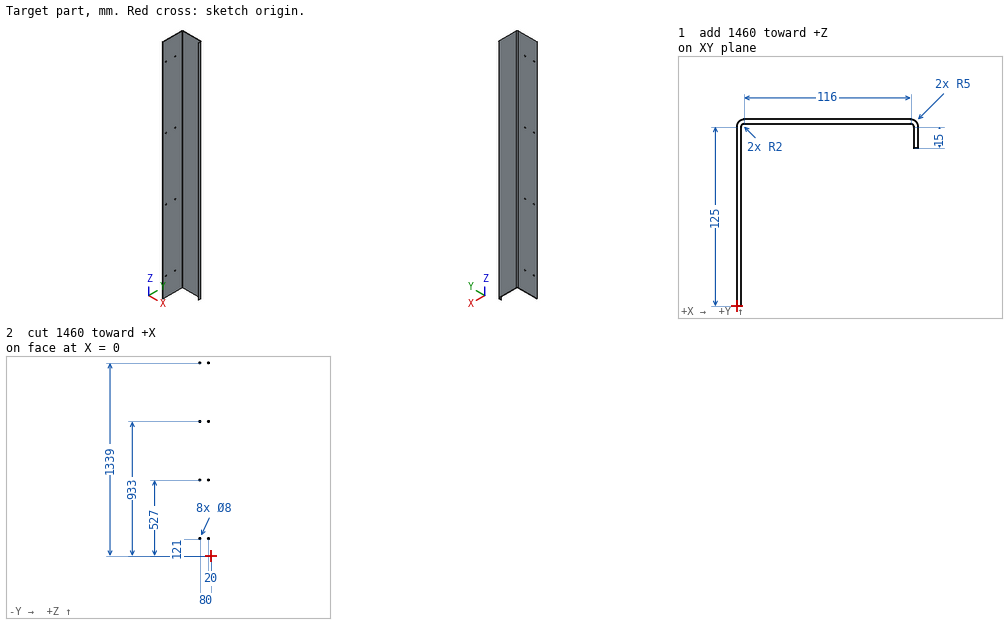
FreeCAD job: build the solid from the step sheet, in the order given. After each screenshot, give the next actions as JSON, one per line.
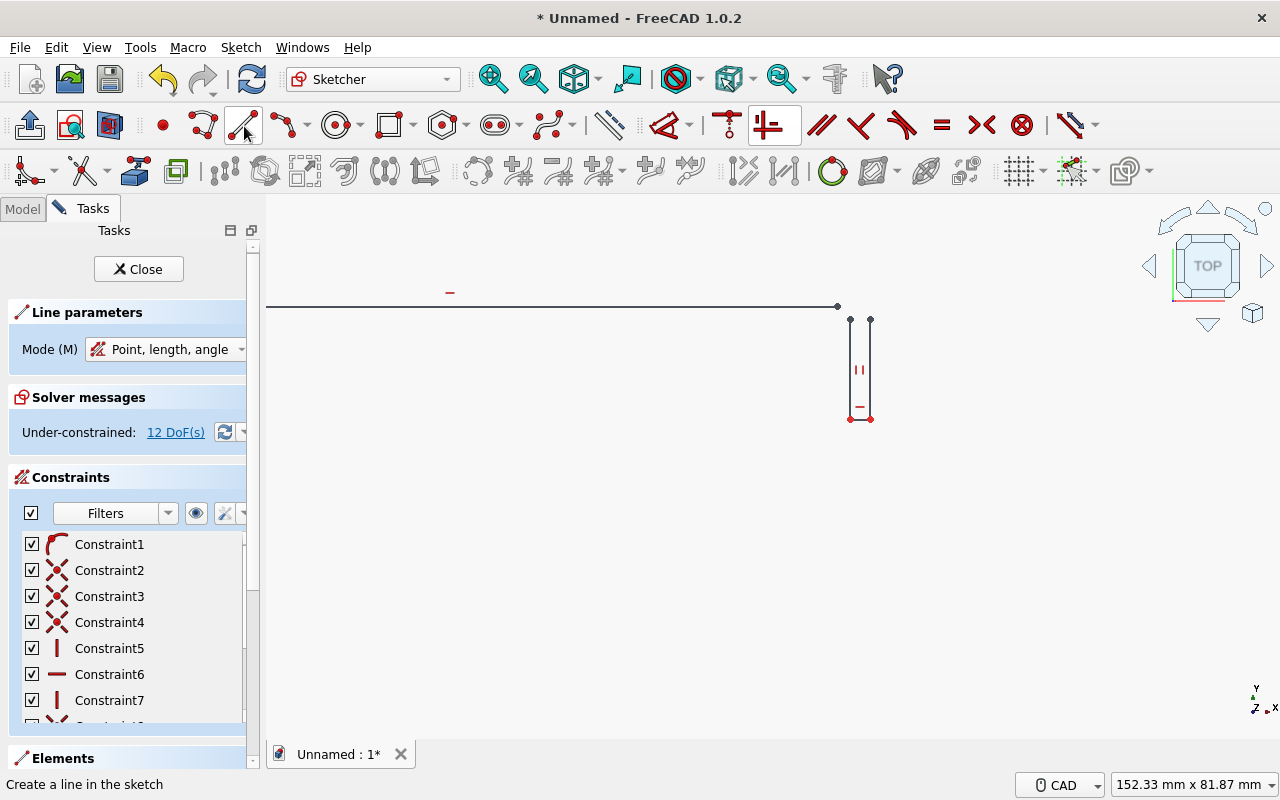
{"action": "left_click", "coordinate": [837, 286]}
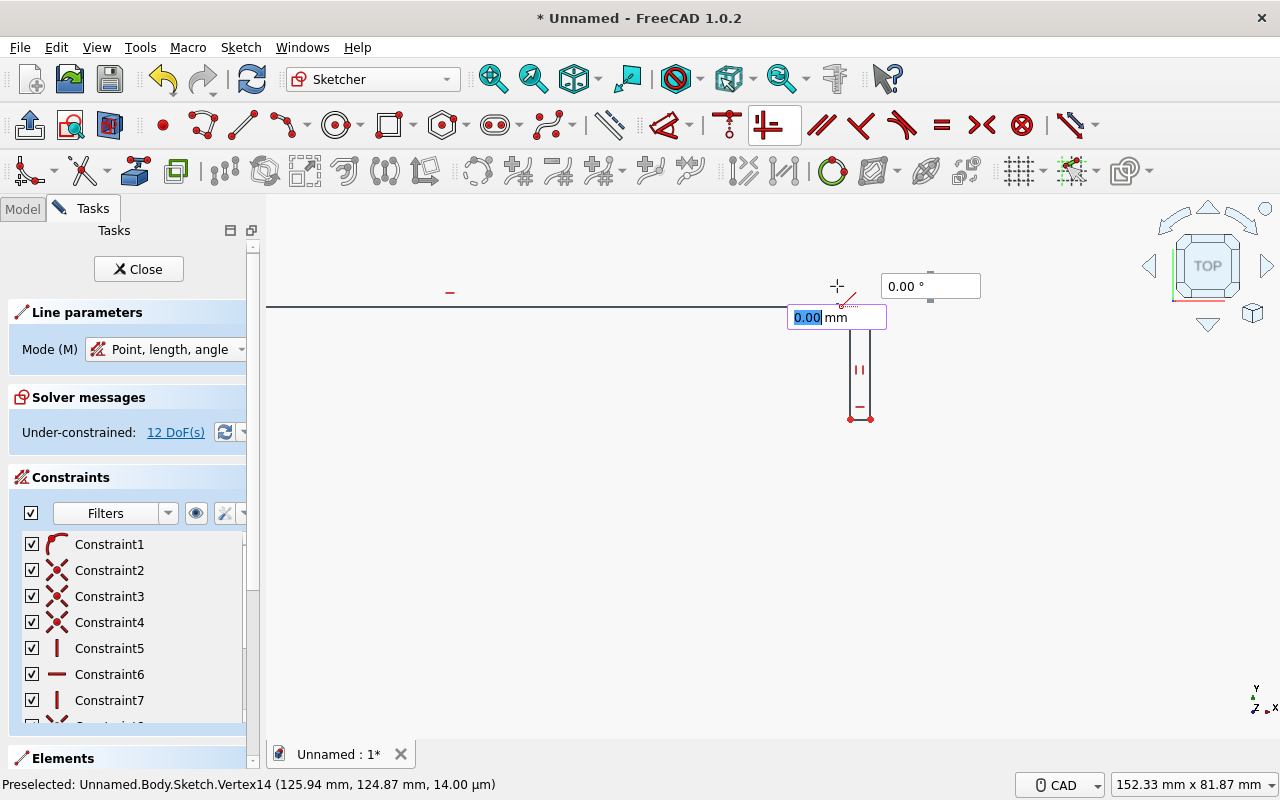
{"action": "scroll", "coordinate": [852, 320], "scroll_direction": "down", "scroll_amount": 5}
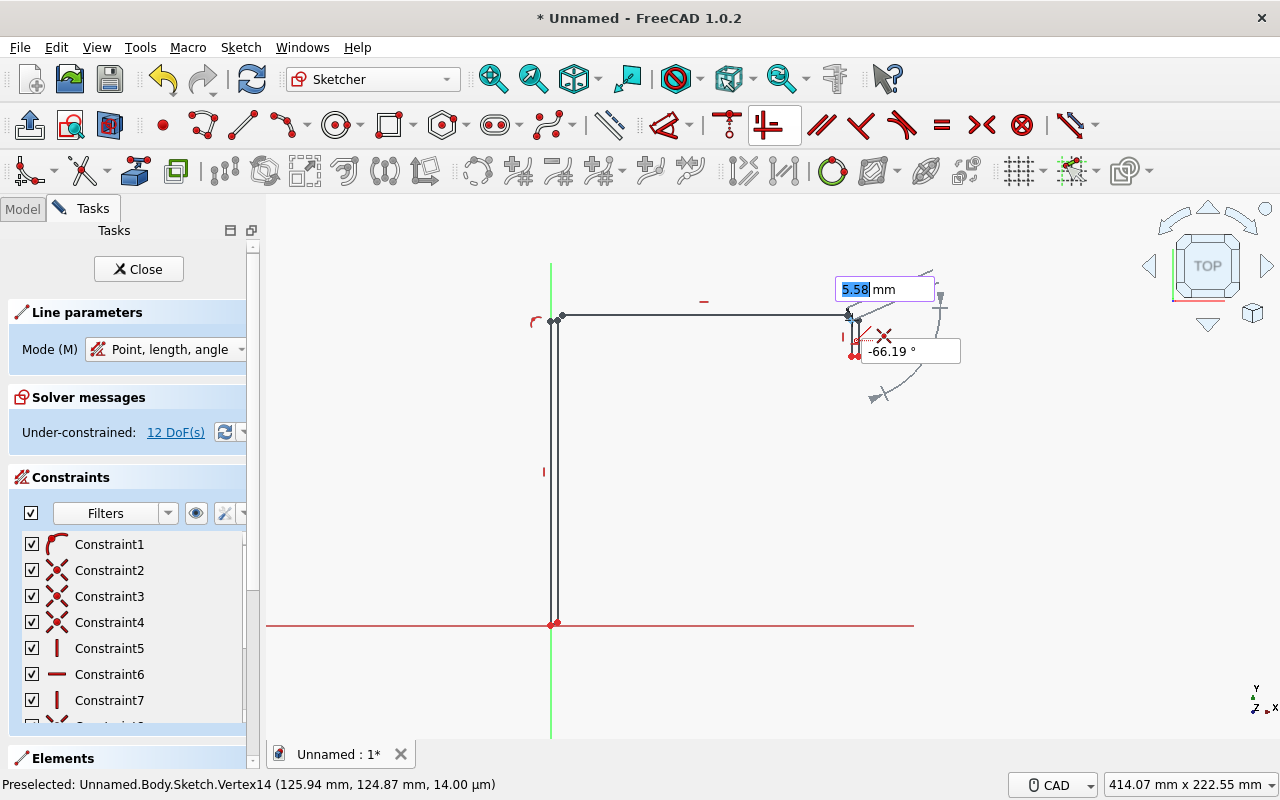
{"action": "scroll", "coordinate": [563, 308], "scroll_direction": "up", "scroll_amount": 4}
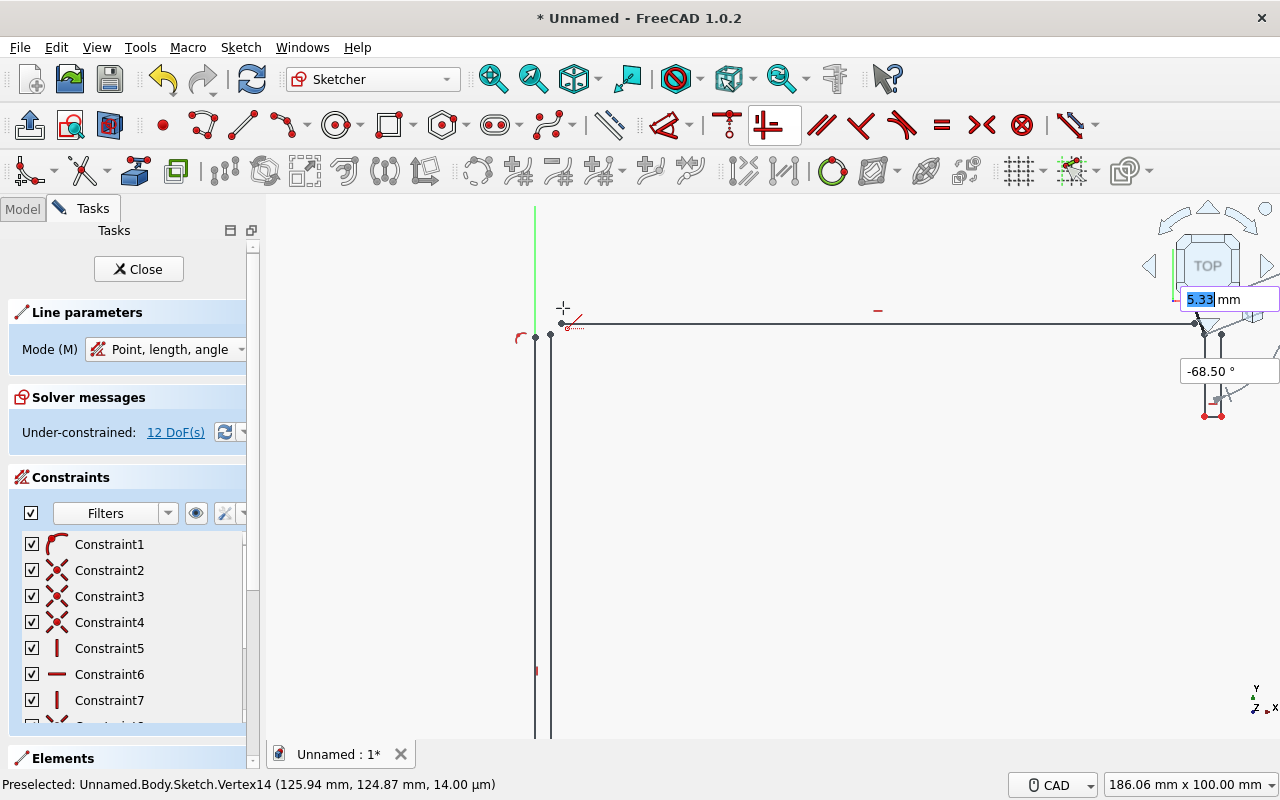
{"action": "left_click", "coordinate": [562, 307]}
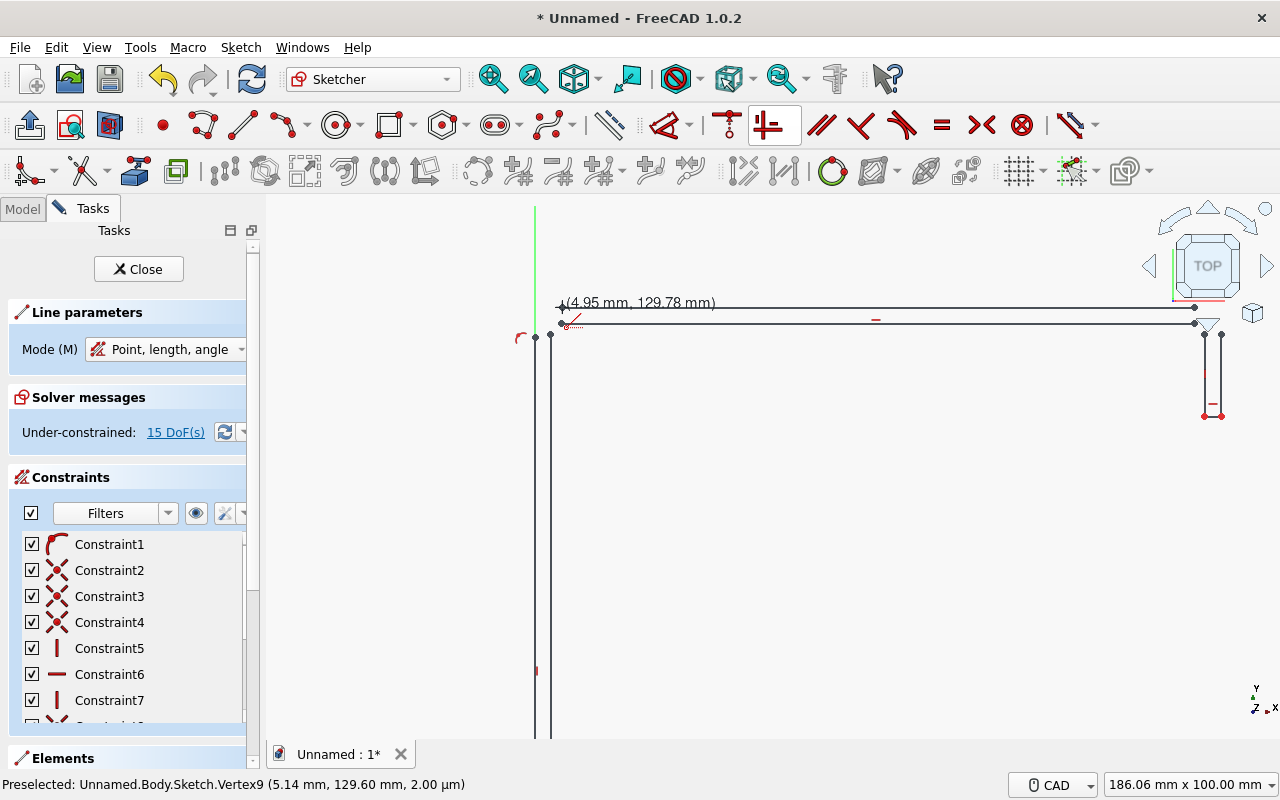
{"action": "left_click", "coordinate": [284, 126]}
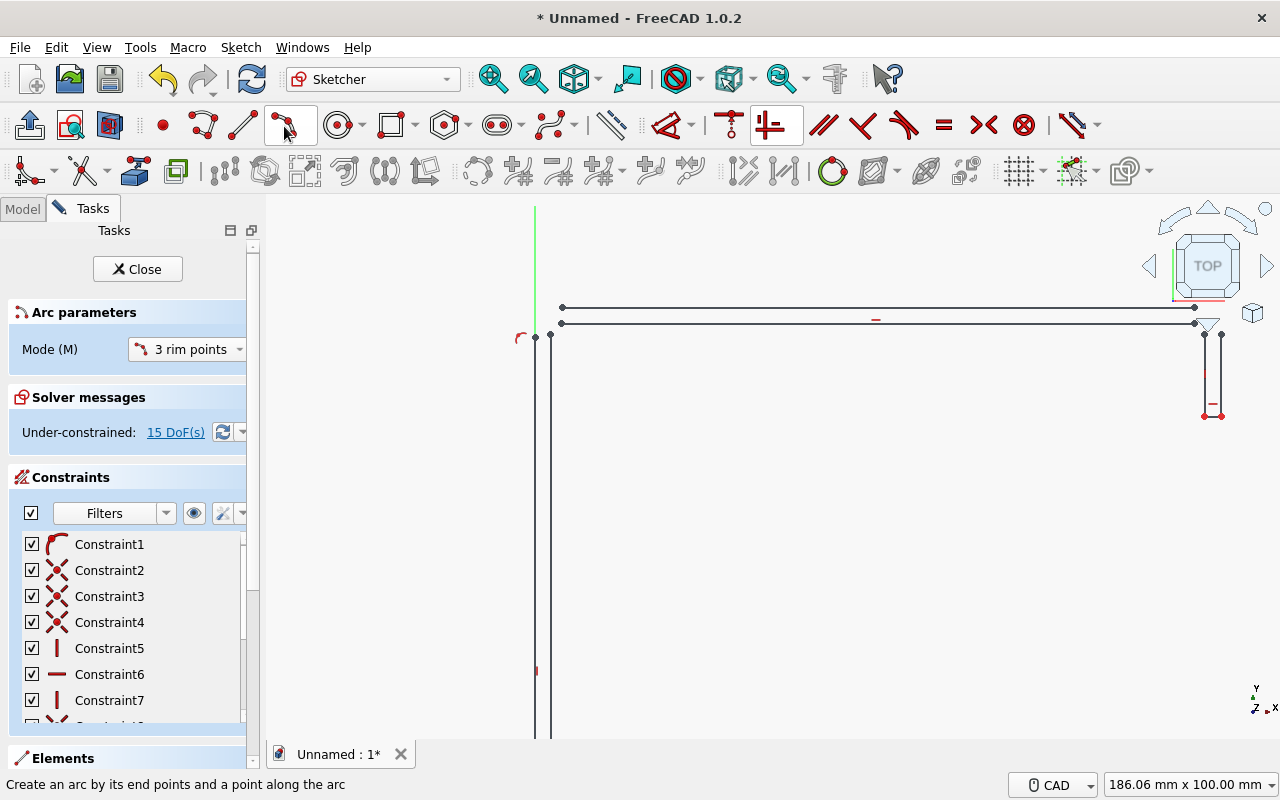
{"action": "left_click", "coordinate": [551, 335]}
{"action": "left_click", "coordinate": [562, 324]}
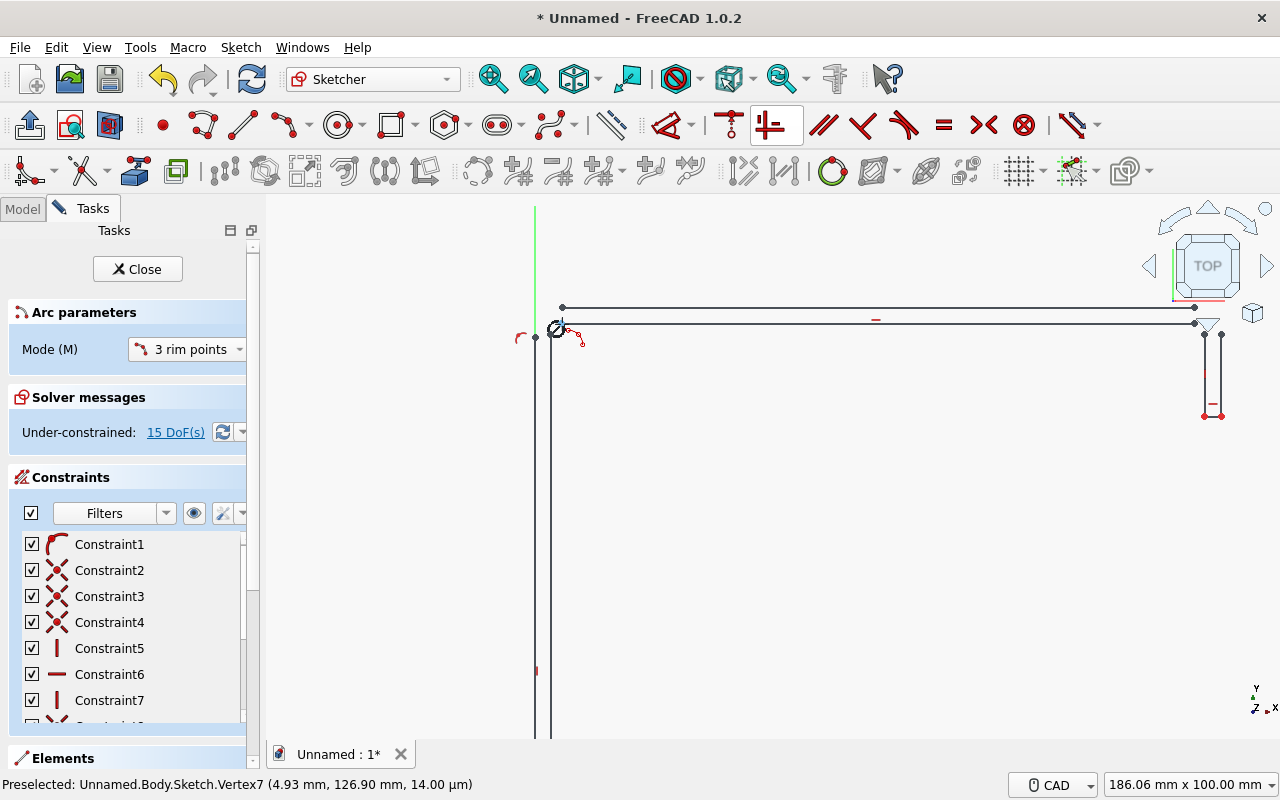
{"action": "scroll", "coordinate": [555, 326], "scroll_direction": "up", "scroll_amount": 9}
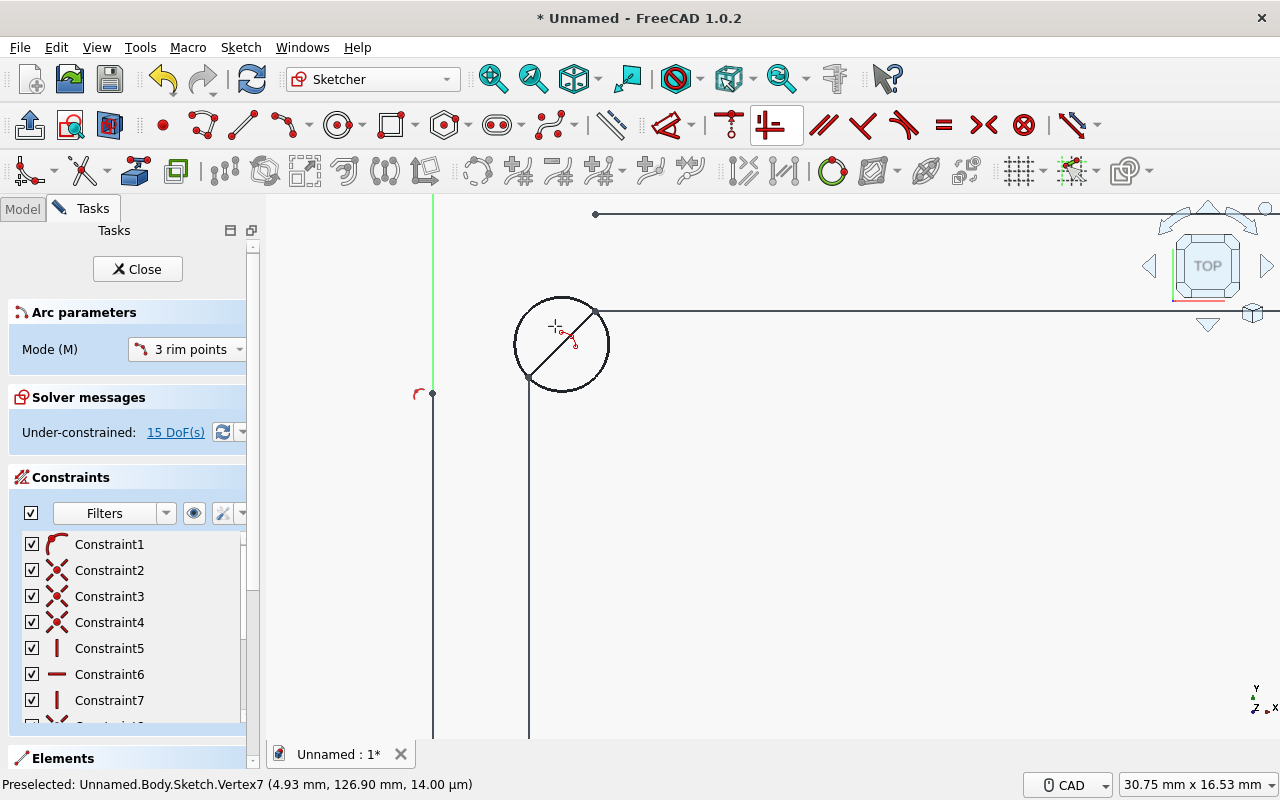
{"action": "left_click", "coordinate": [551, 327]}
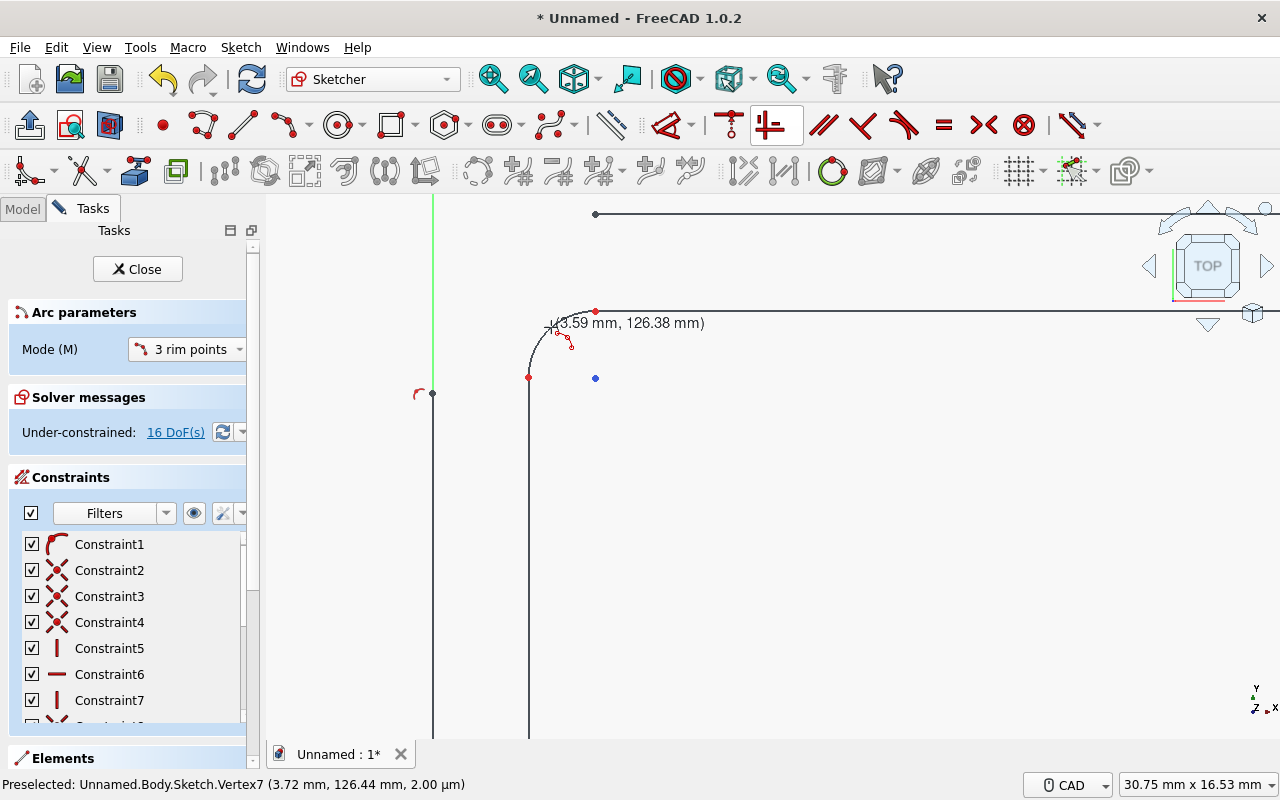
{"action": "scroll", "coordinate": [560, 315], "scroll_direction": "down", "scroll_amount": 13}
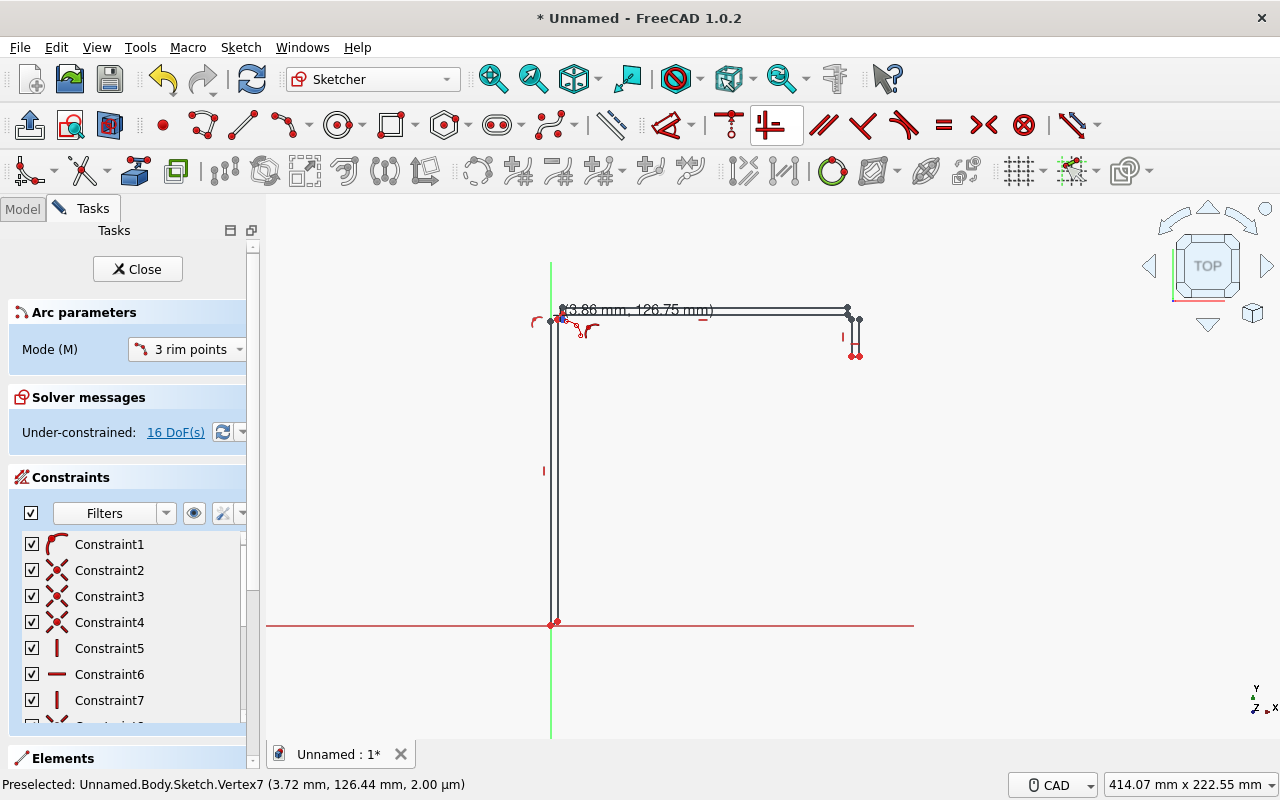
{"action": "scroll", "coordinate": [847, 315], "scroll_direction": "up", "scroll_amount": 5}